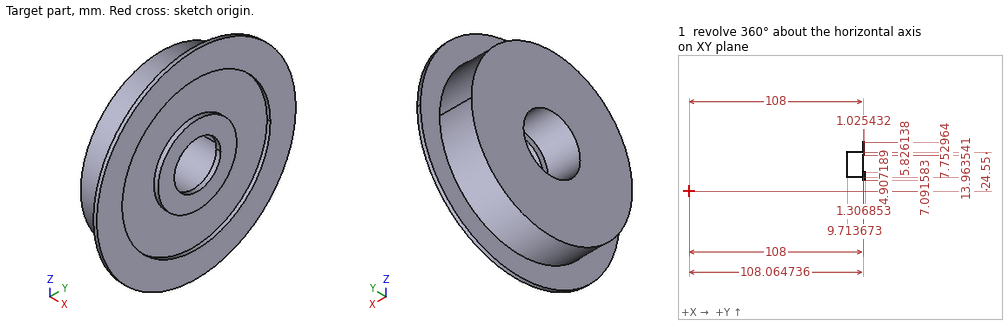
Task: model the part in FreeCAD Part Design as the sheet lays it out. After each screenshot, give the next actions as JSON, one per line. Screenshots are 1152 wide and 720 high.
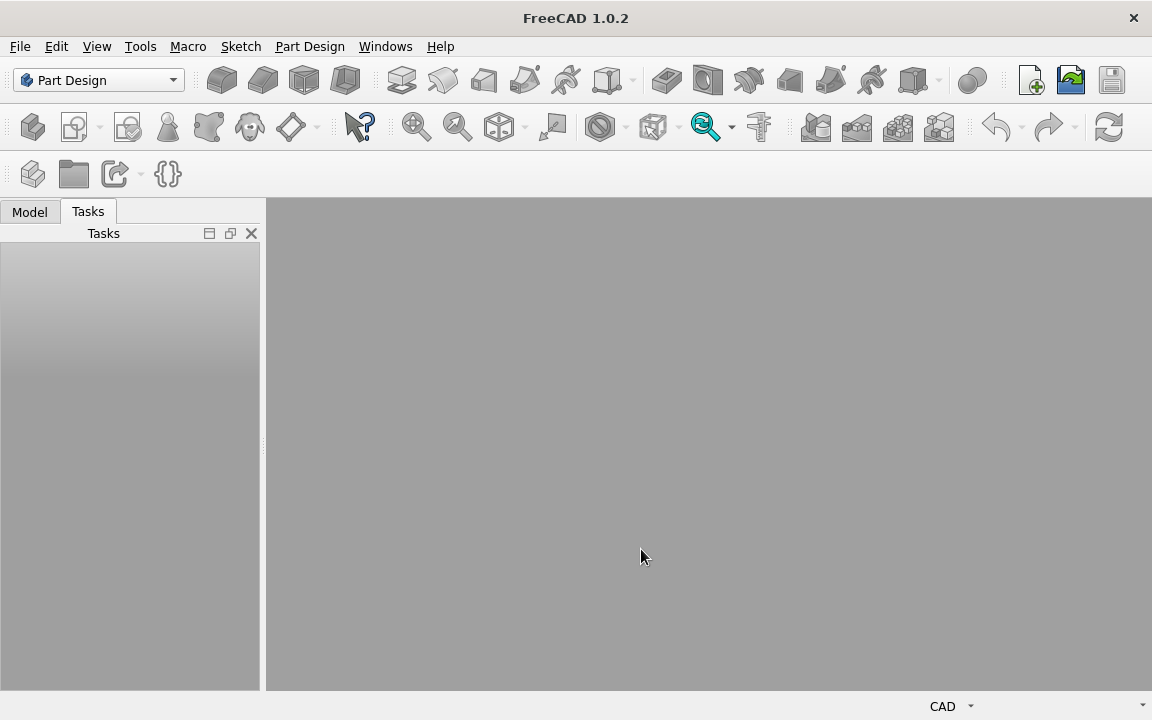
{"action": "left_click", "coordinate": [1030, 80]}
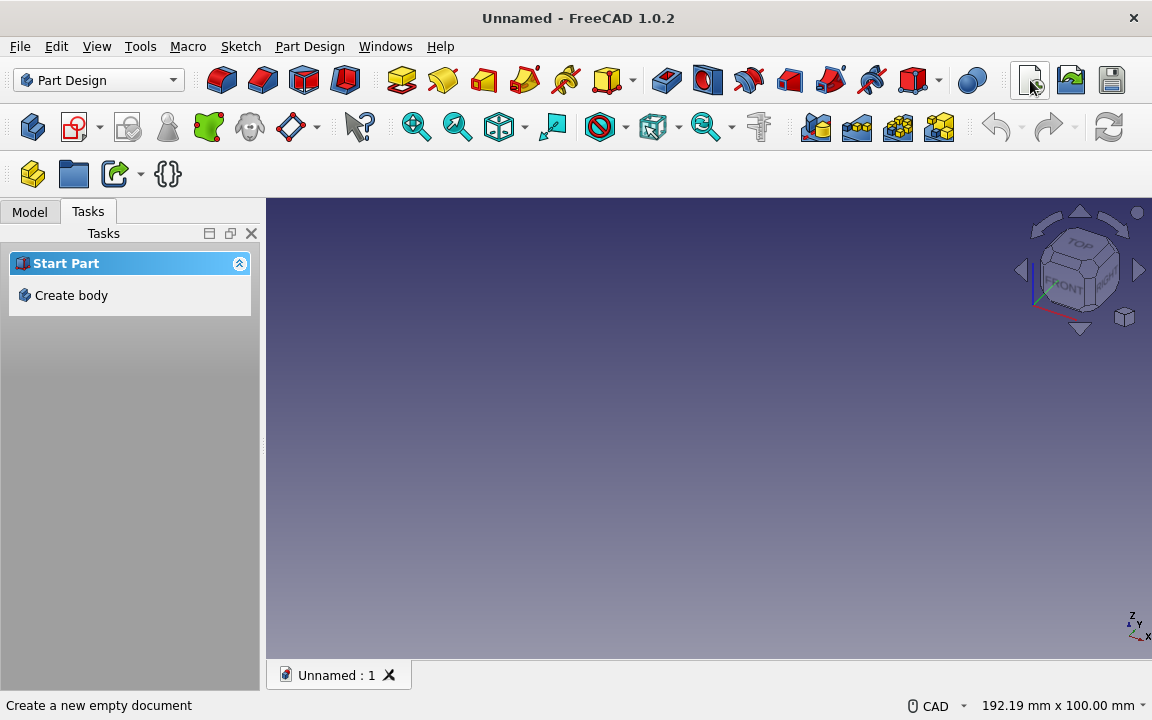
{"action": "left_click", "coordinate": [33, 128]}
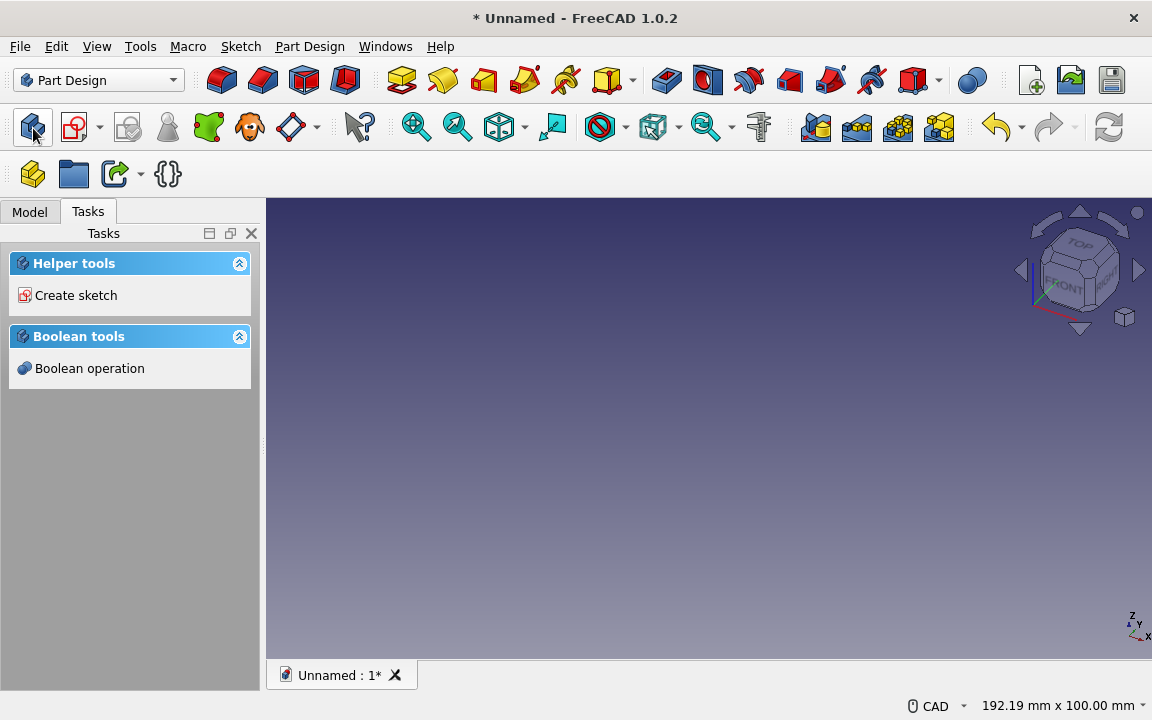
{"action": "left_click", "coordinate": [30, 212]}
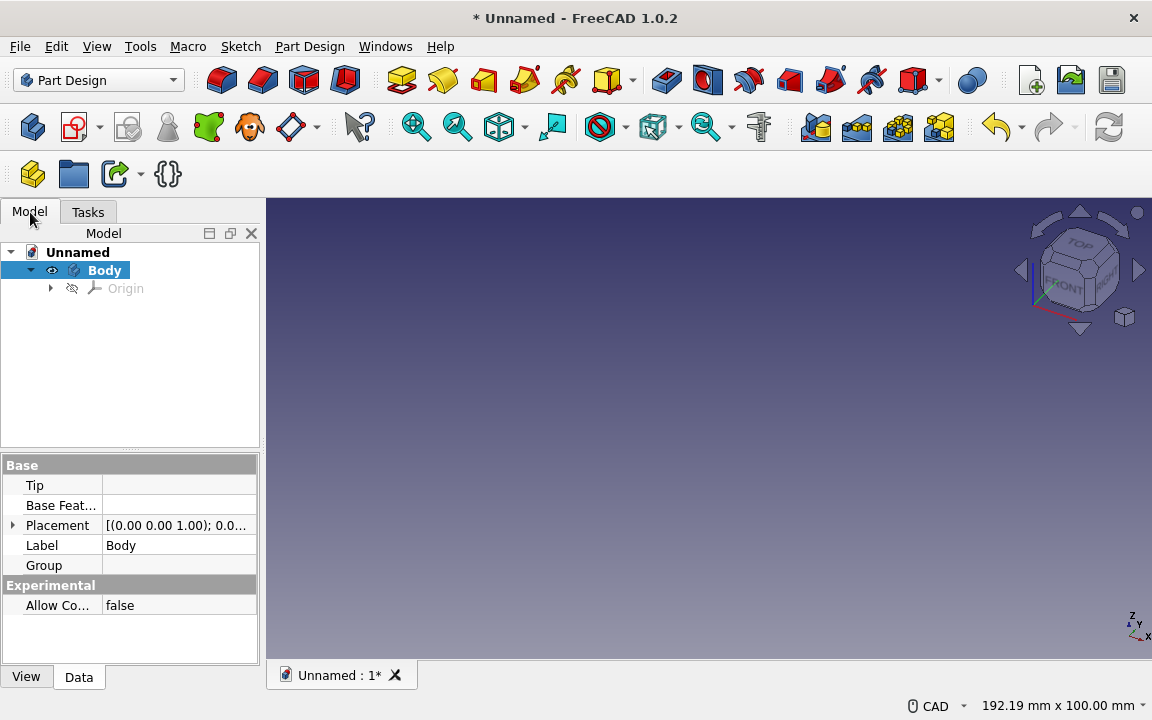
{"action": "left_click", "coordinate": [97, 270]}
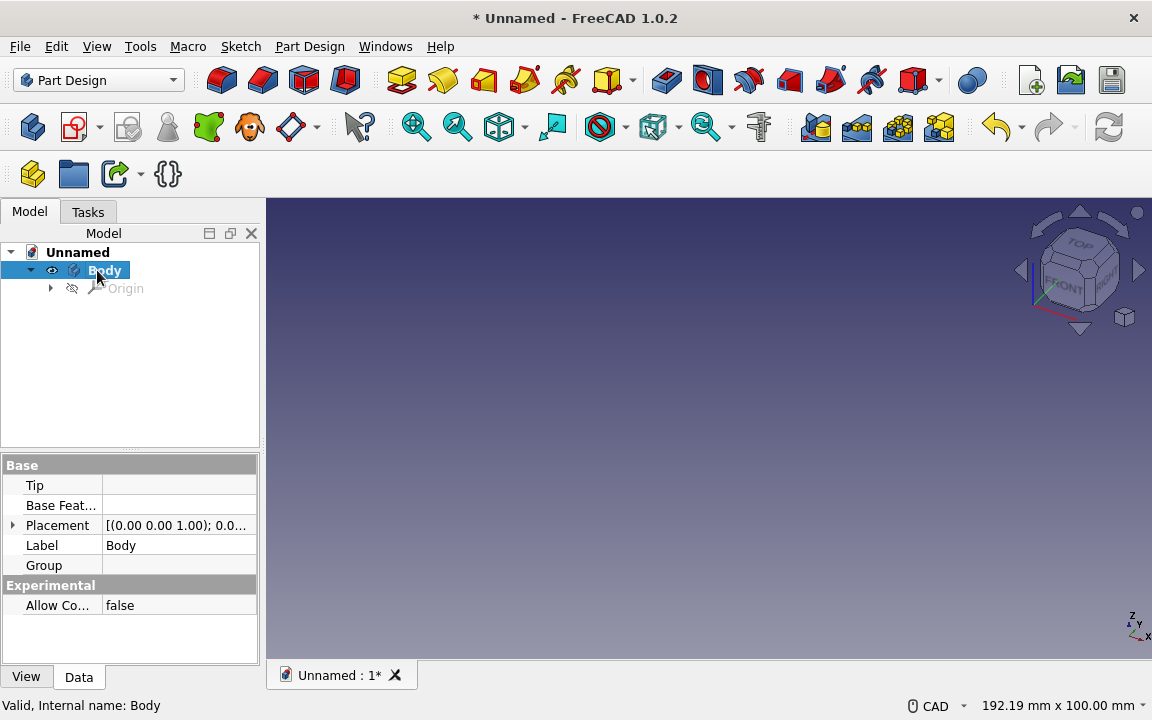
{"action": "left_click", "coordinate": [148, 605]}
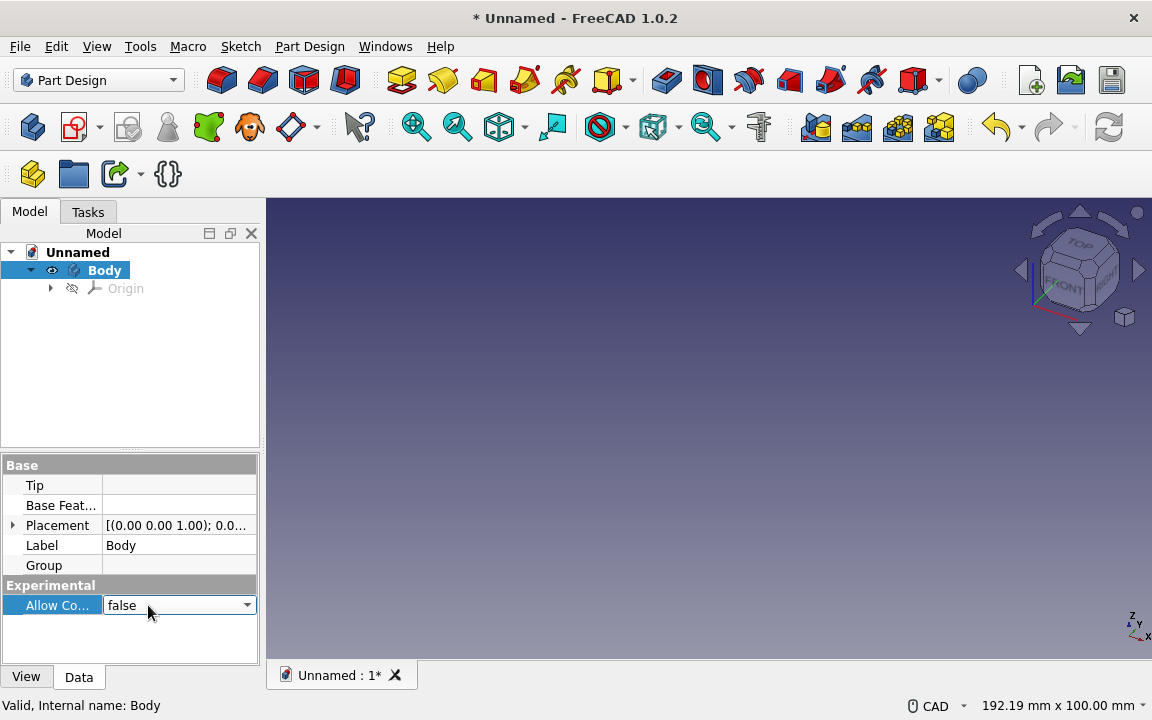
{"action": "left_click", "coordinate": [148, 605]}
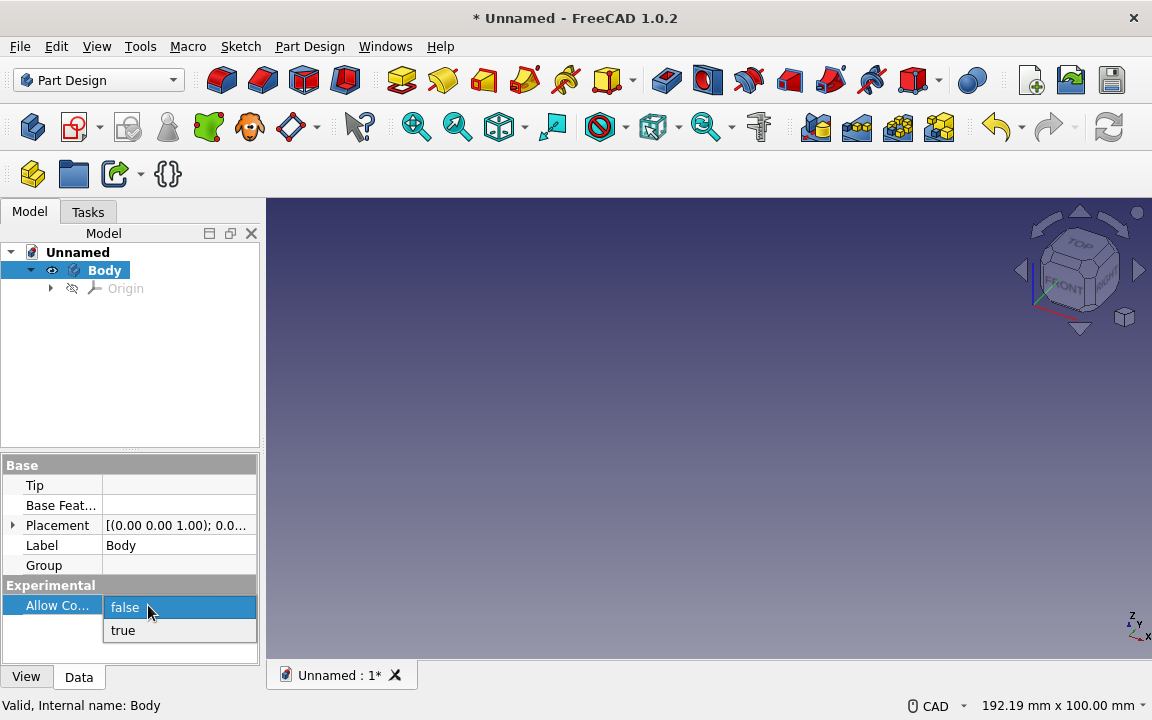
{"action": "left_click", "coordinate": [178, 630]}
{"action": "key", "text": "Return"}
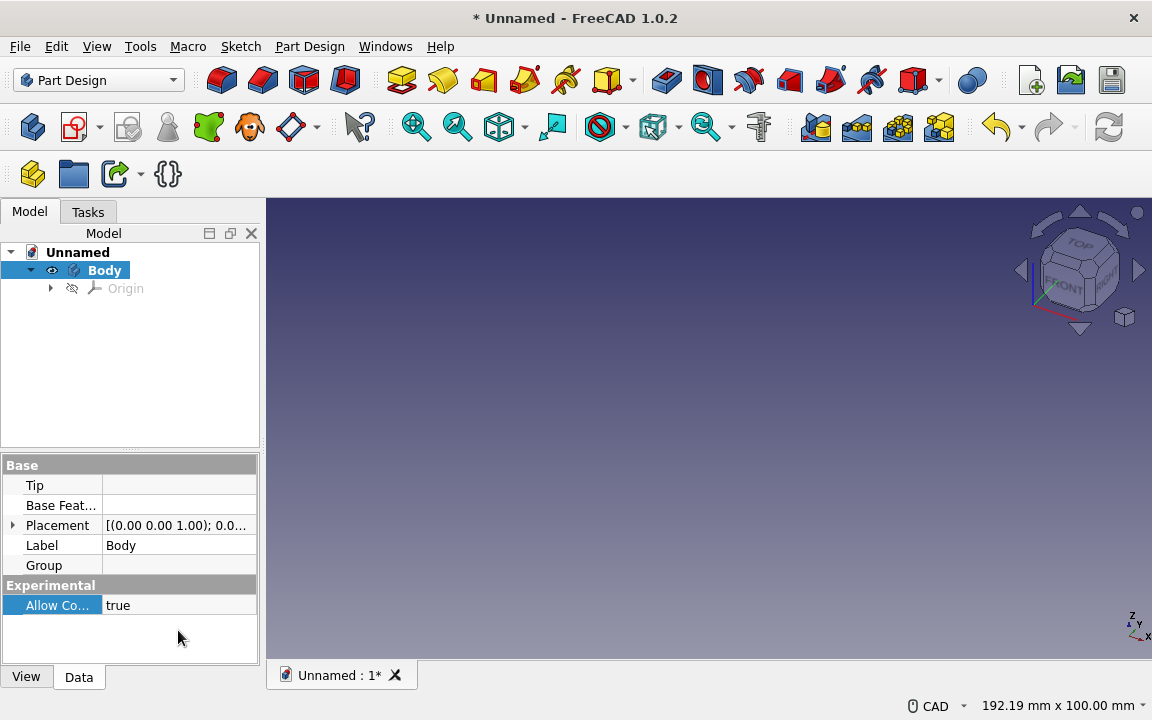
{"action": "left_click", "coordinate": [306, 619]}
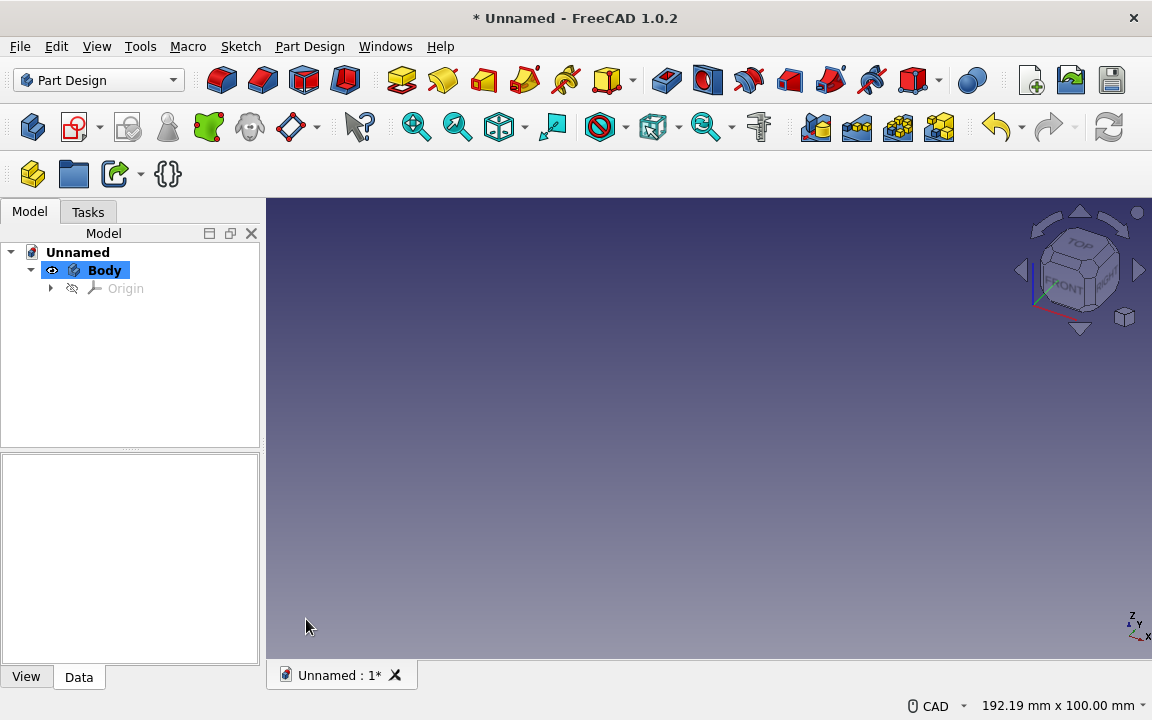
{"action": "left_click", "coordinate": [74, 128]}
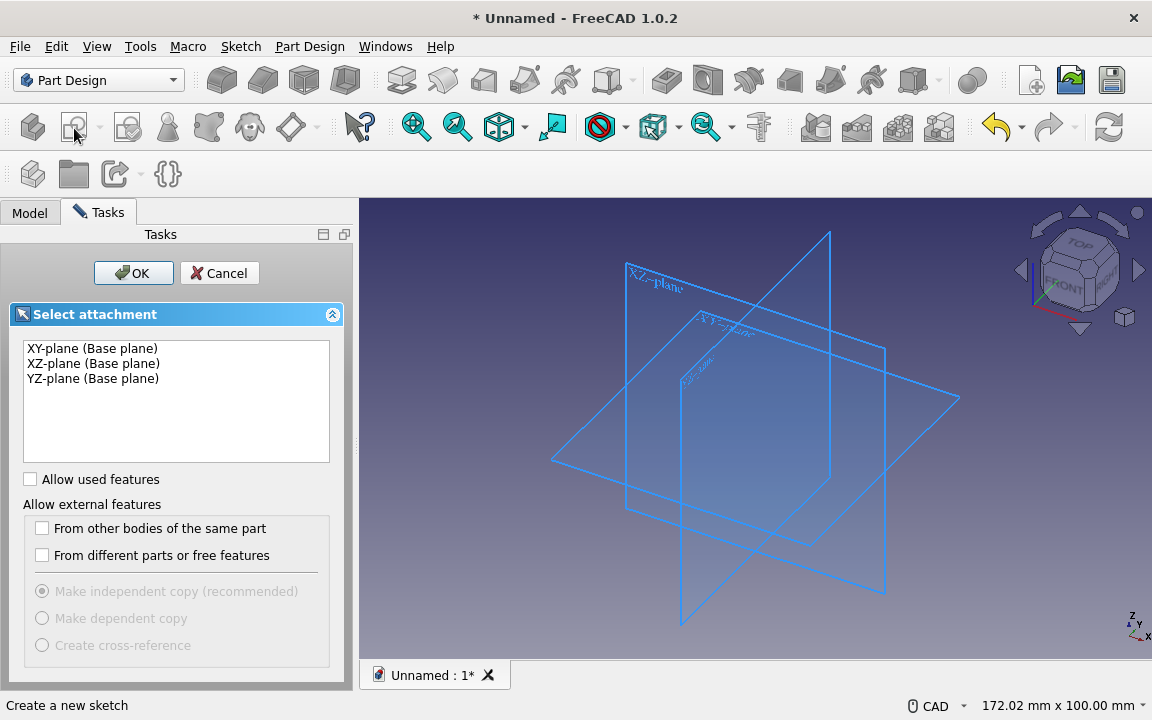
{"action": "left_click", "coordinate": [84, 348]}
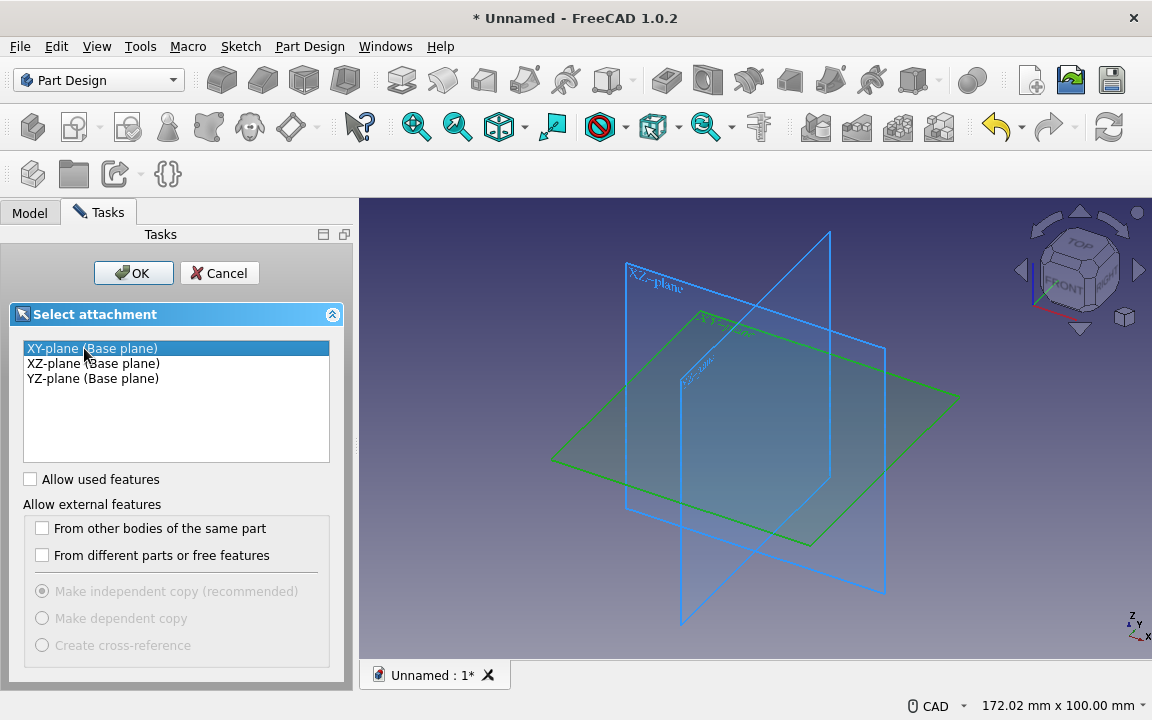
{"action": "left_click", "coordinate": [134, 273]}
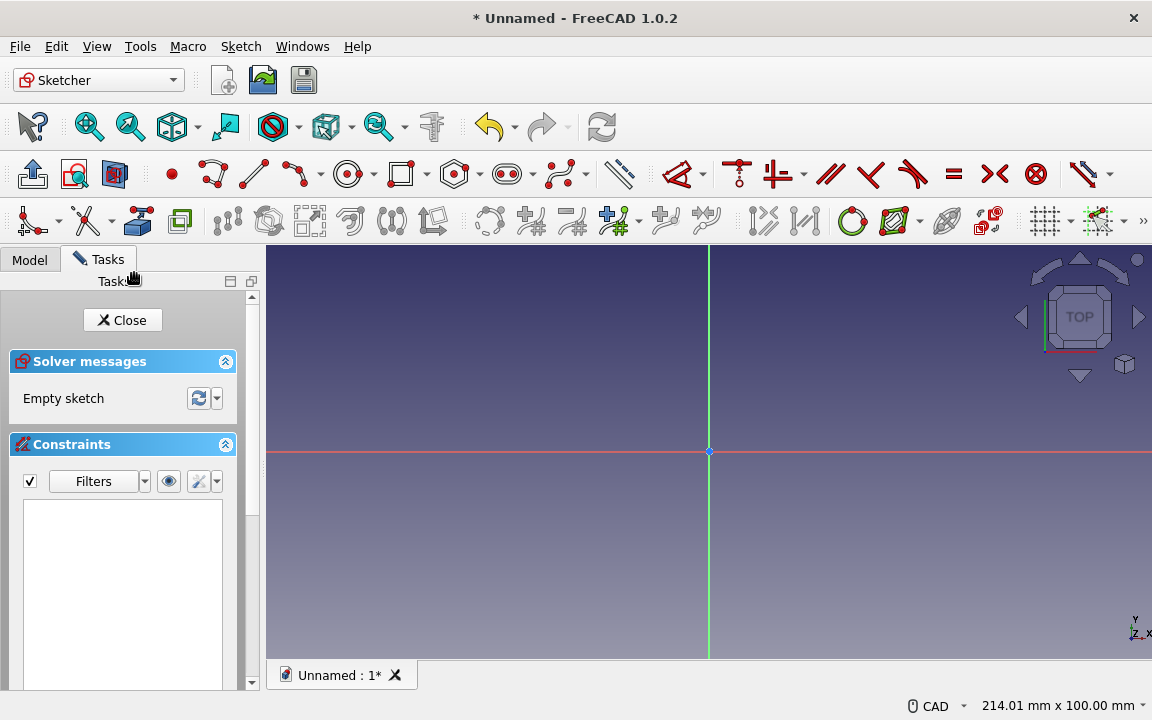
{"action": "scroll", "coordinate": [640, 452], "scroll_direction": "down", "scroll_amount": 5}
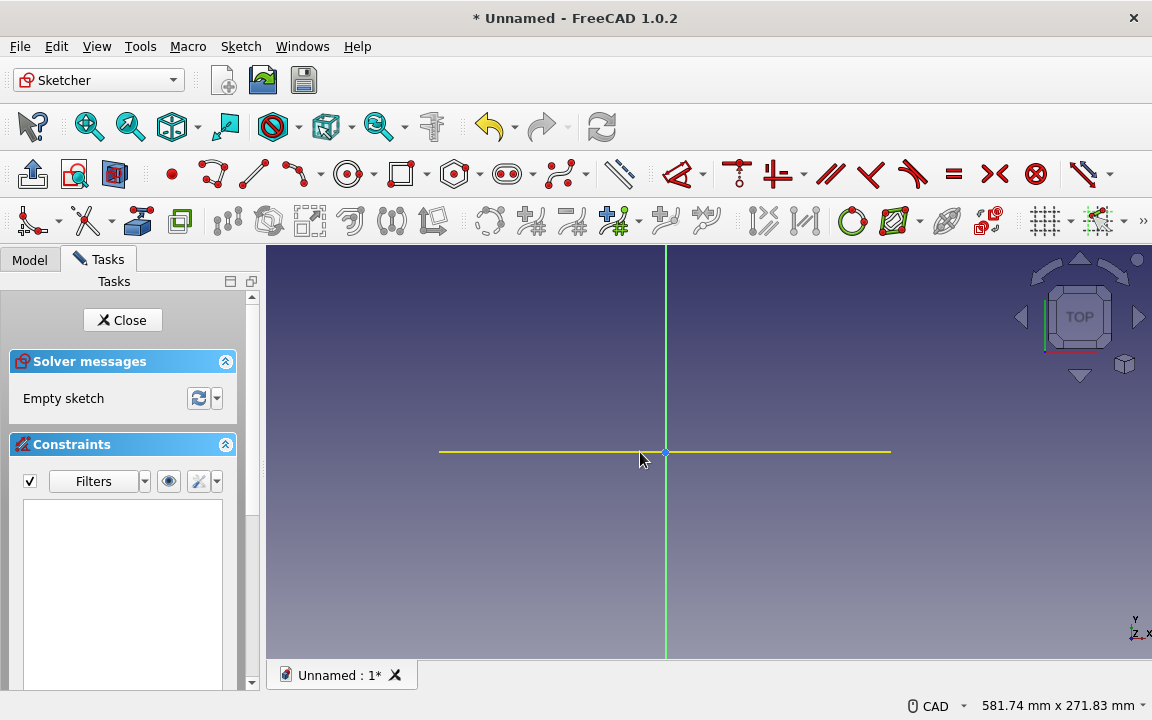
{"action": "scroll", "coordinate": [852, 419], "scroll_direction": "up", "scroll_amount": 10}